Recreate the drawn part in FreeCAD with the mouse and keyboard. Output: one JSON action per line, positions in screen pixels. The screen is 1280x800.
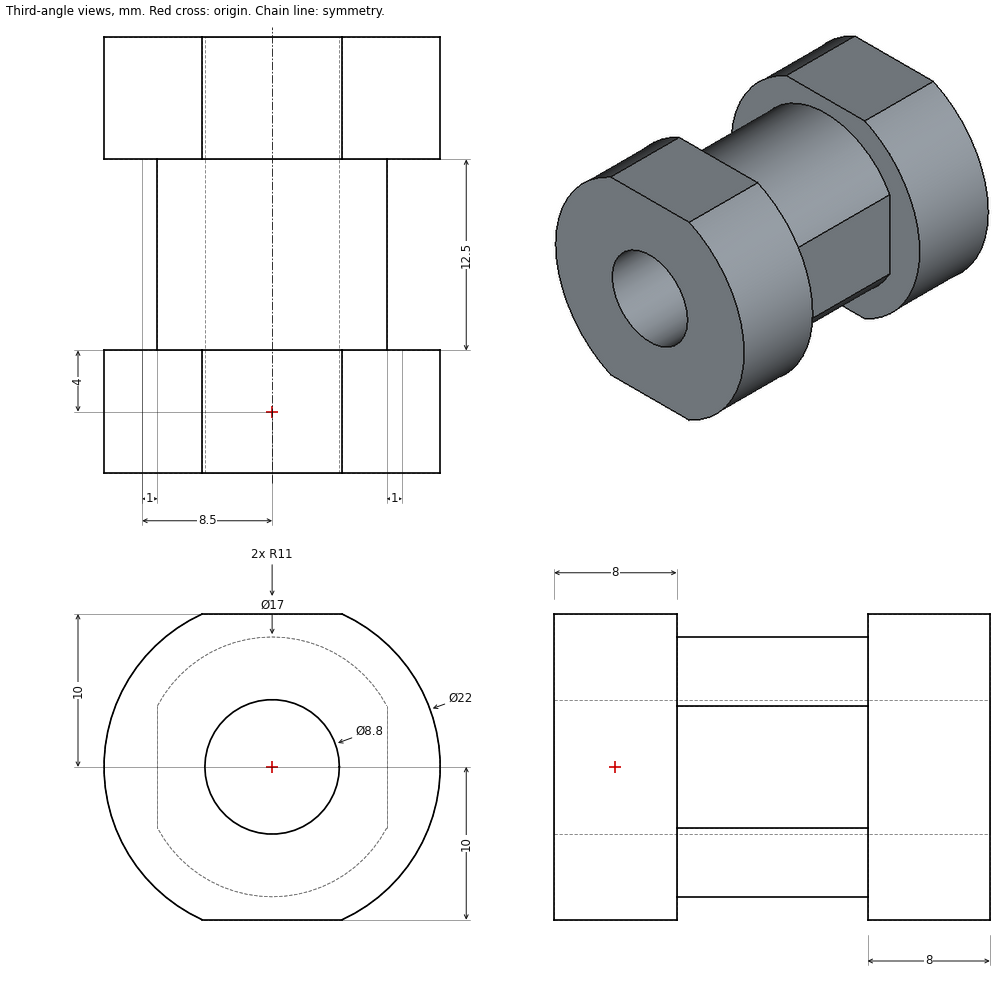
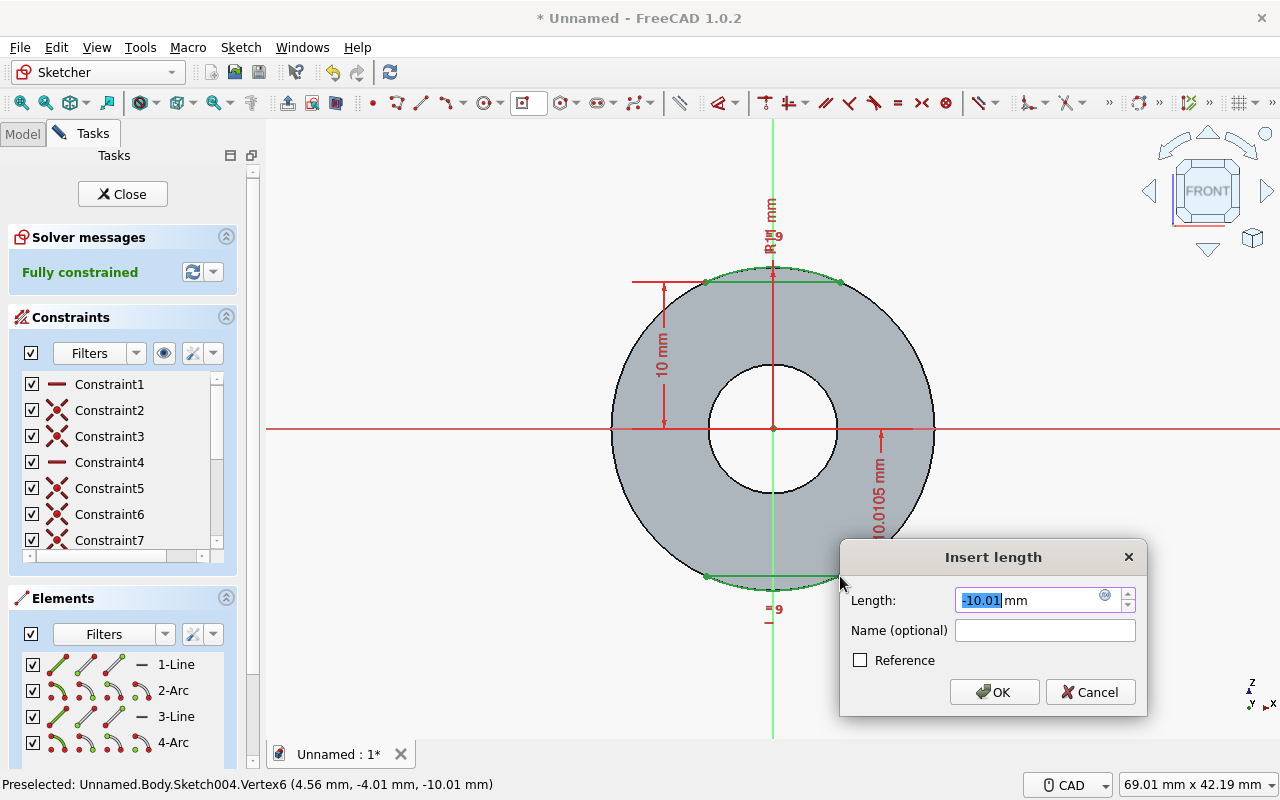
{"action": "type", "text": "-10"}
{"action": "key", "text": "Return"}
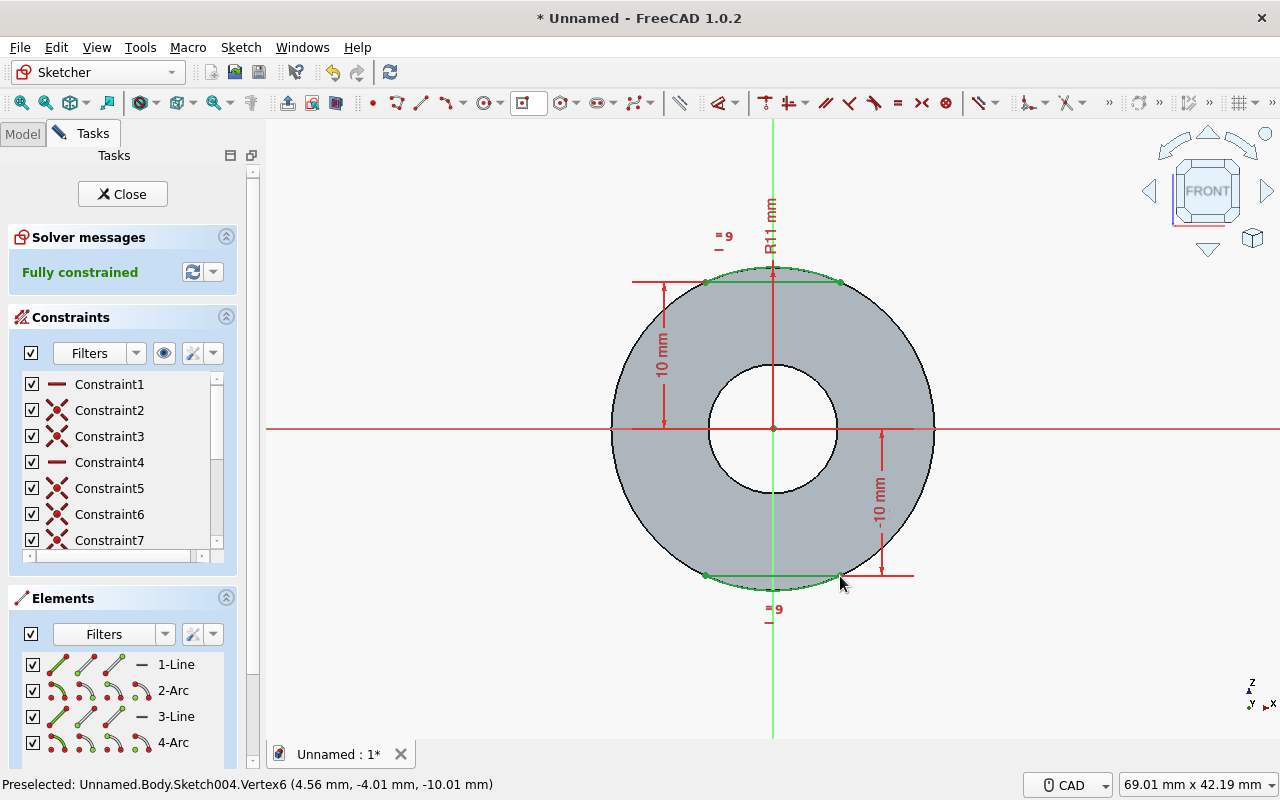
{"action": "left_click", "coordinate": [123, 194]}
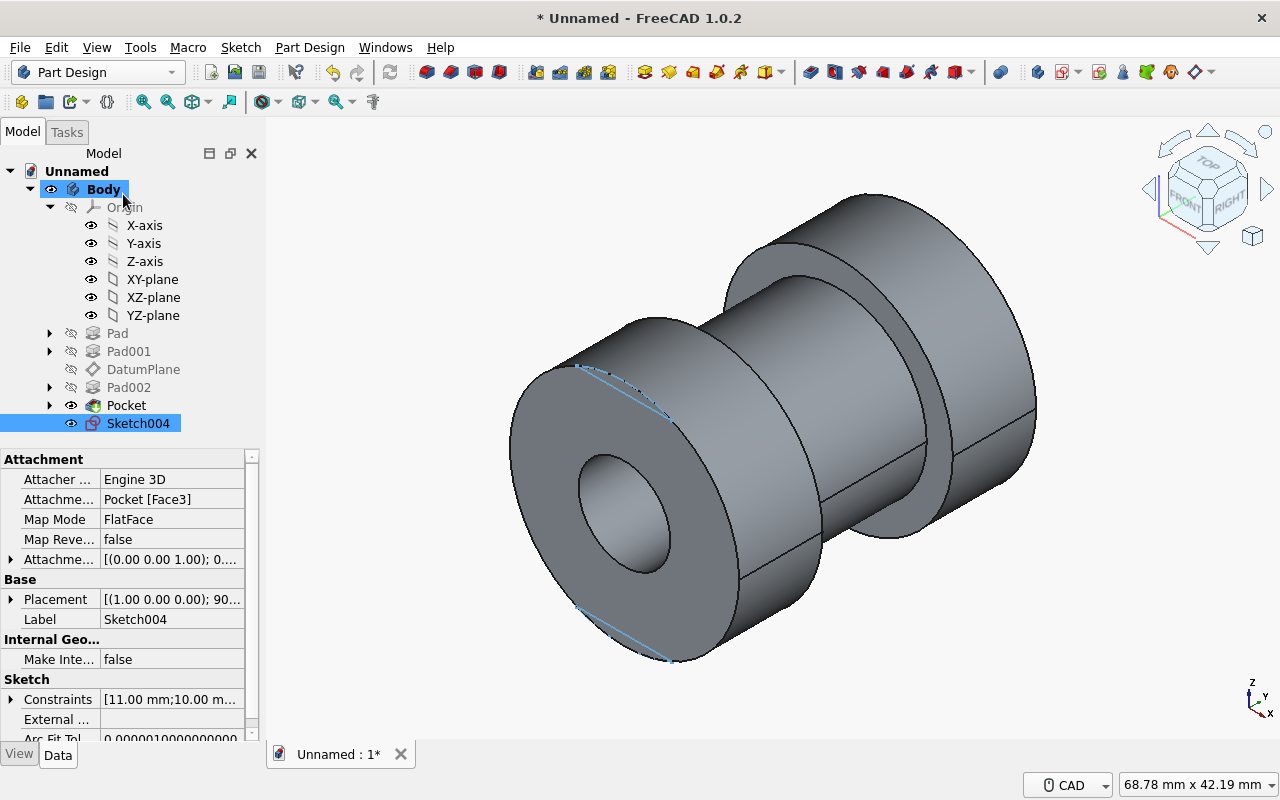
{"action": "left_click", "coordinate": [812, 72]}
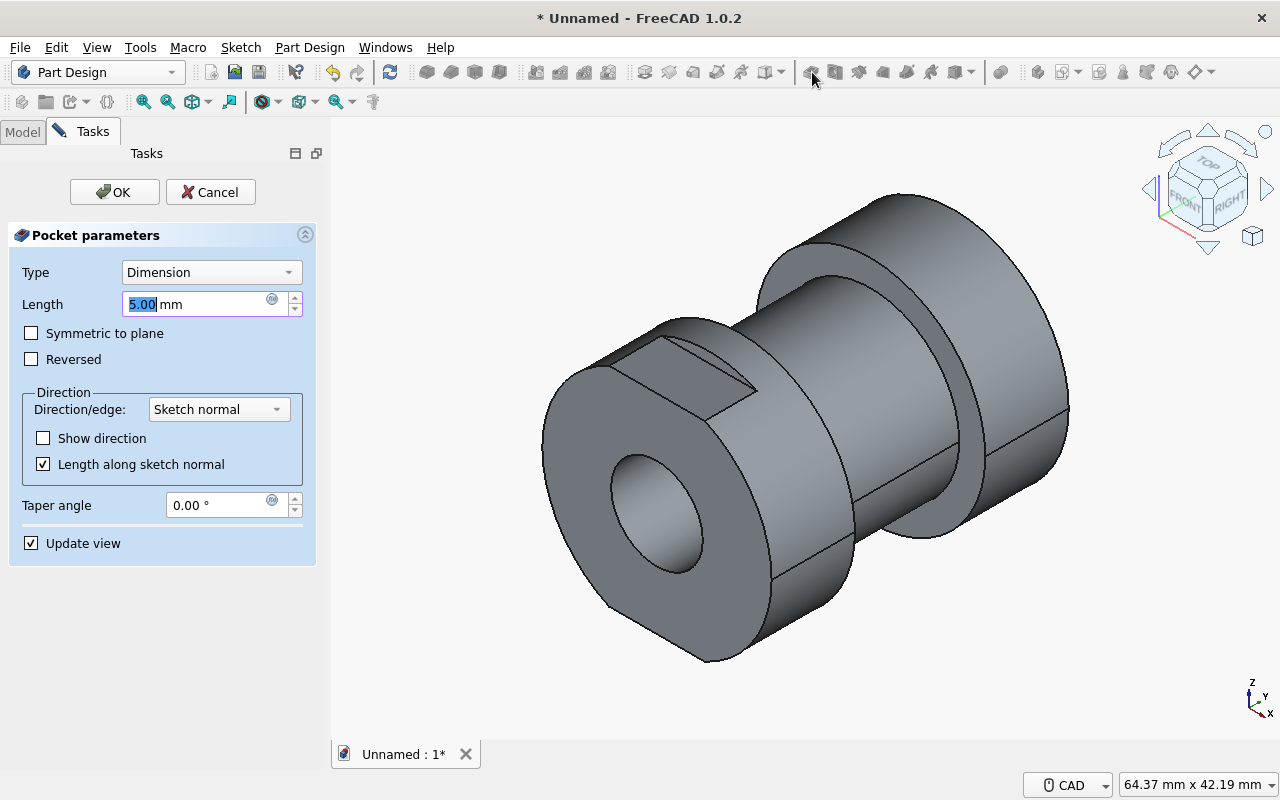
{"action": "left_click", "coordinate": [212, 272]}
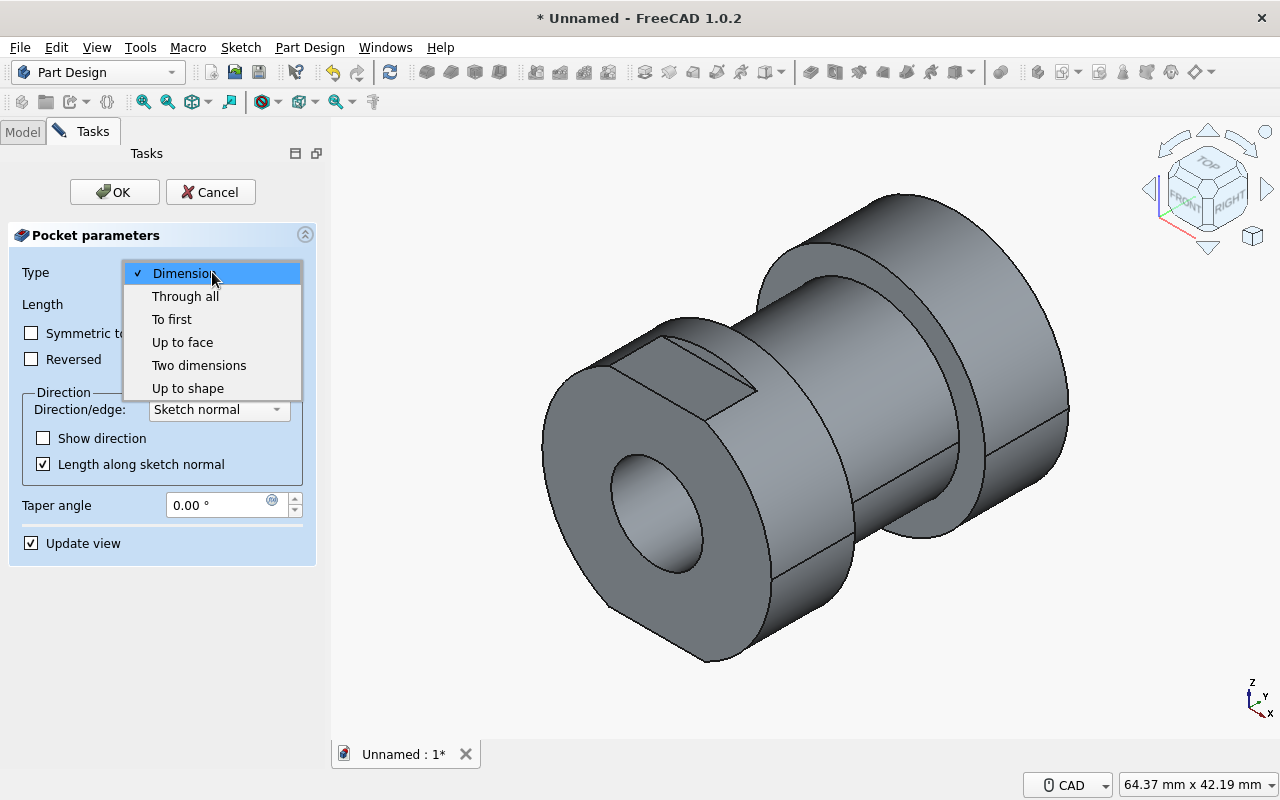
{"action": "left_click", "coordinate": [212, 296]}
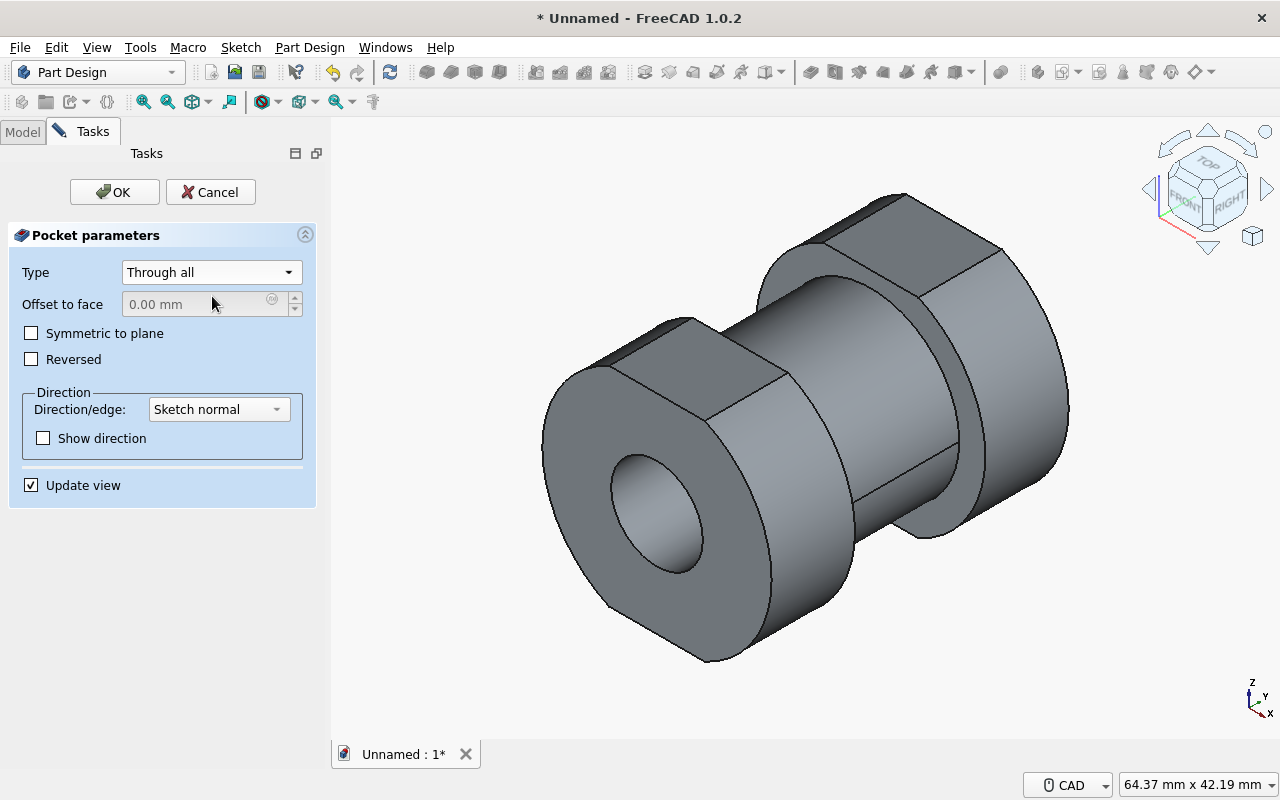
{"action": "left_click", "coordinate": [115, 192]}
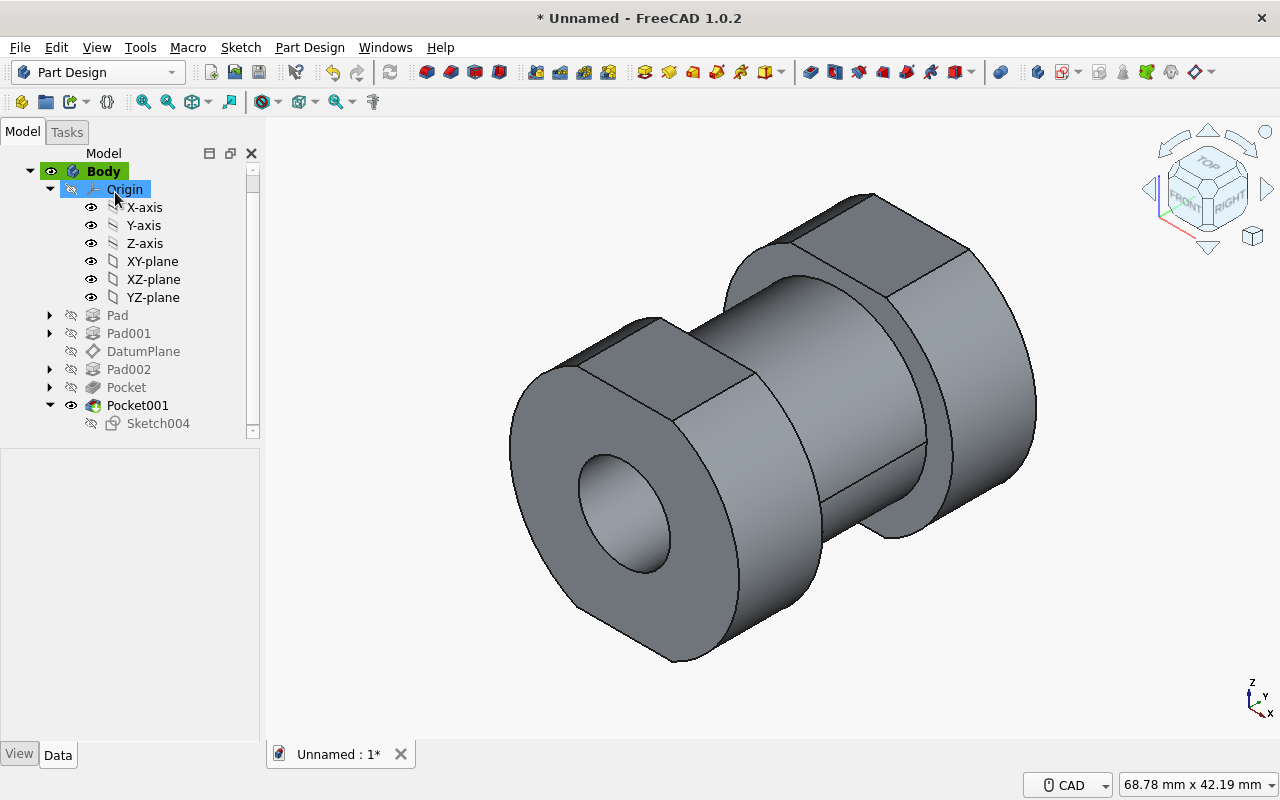
{"action": "left_click", "coordinate": [1062, 72]}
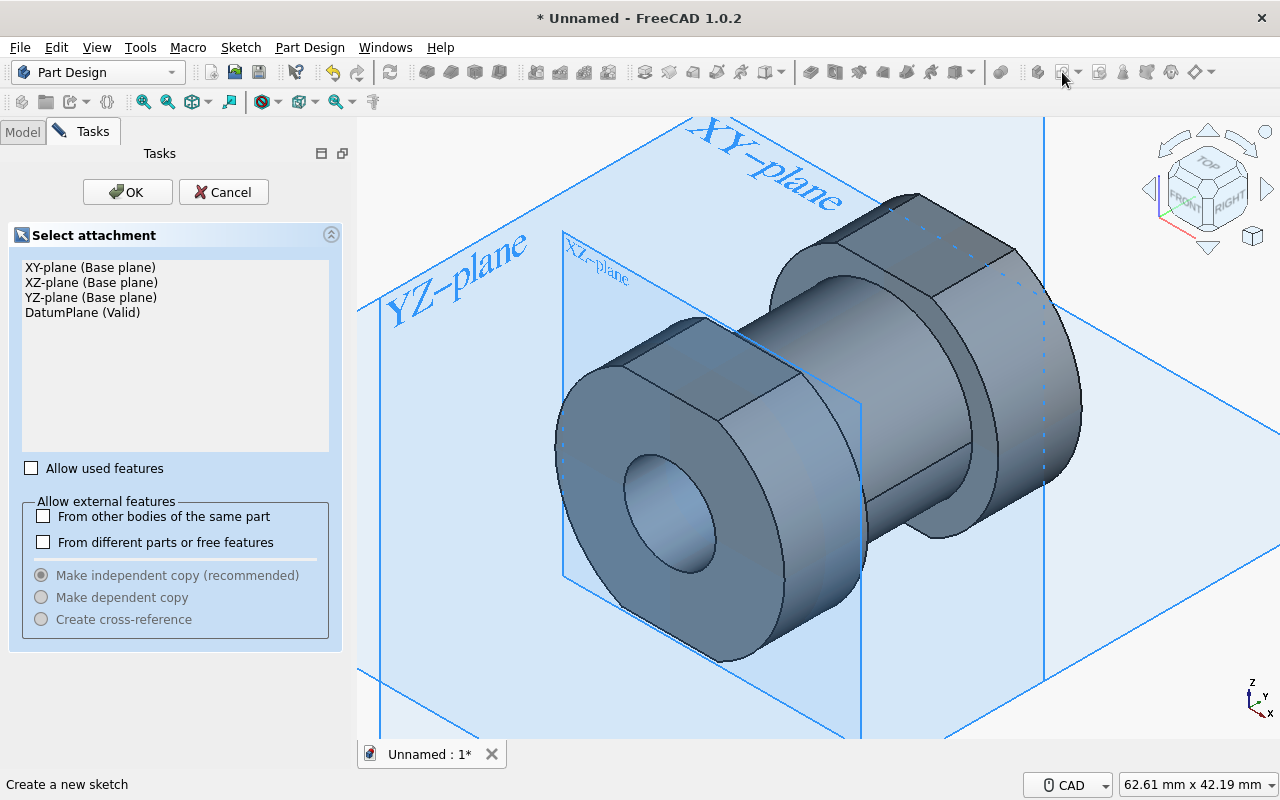
{"action": "left_click", "coordinate": [82, 268]}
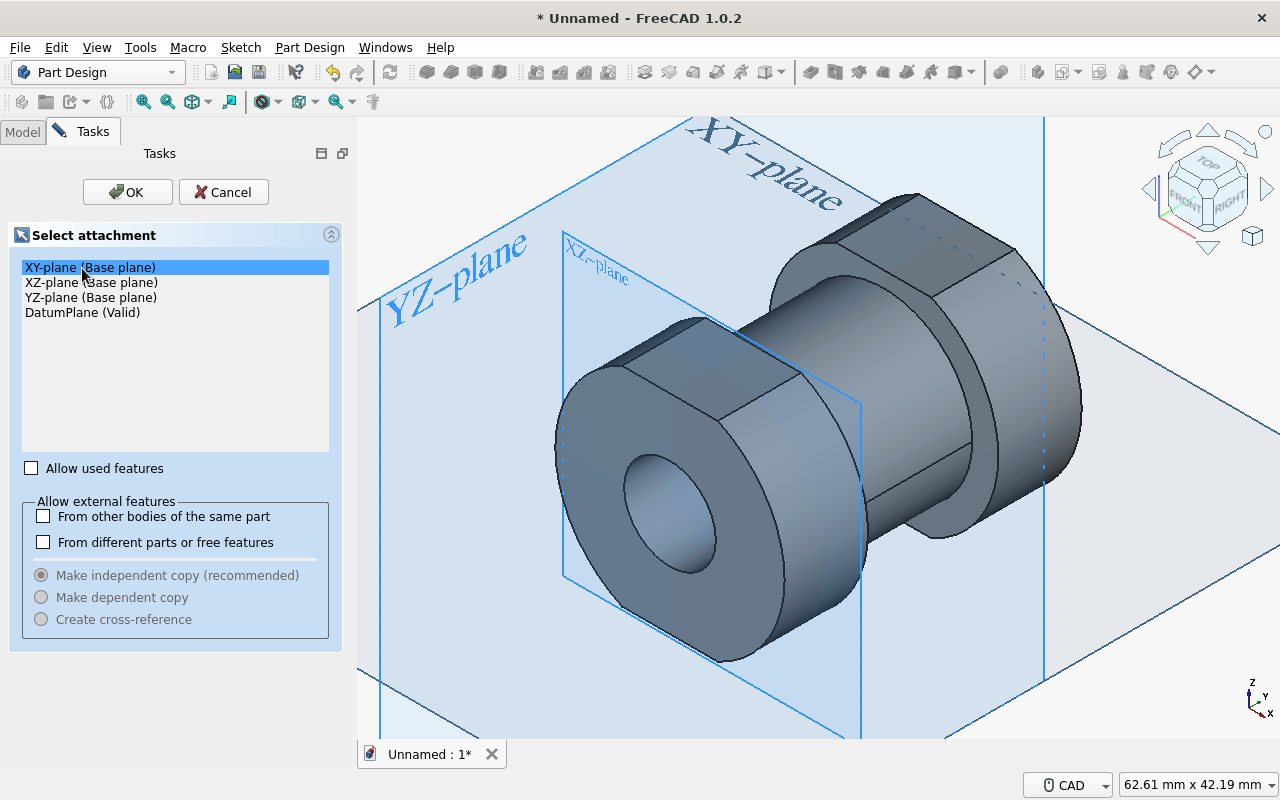
{"action": "left_click", "coordinate": [128, 192]}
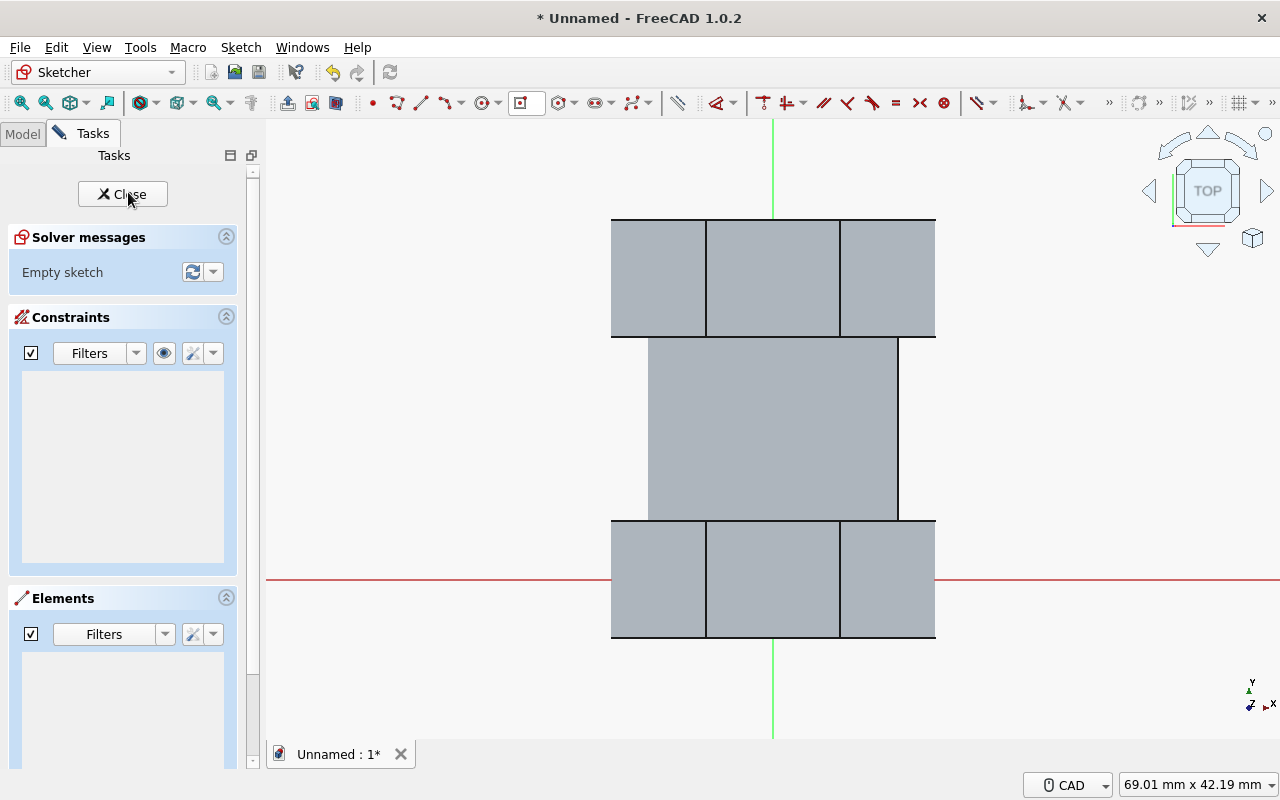
{"action": "left_click", "coordinate": [336, 104]}